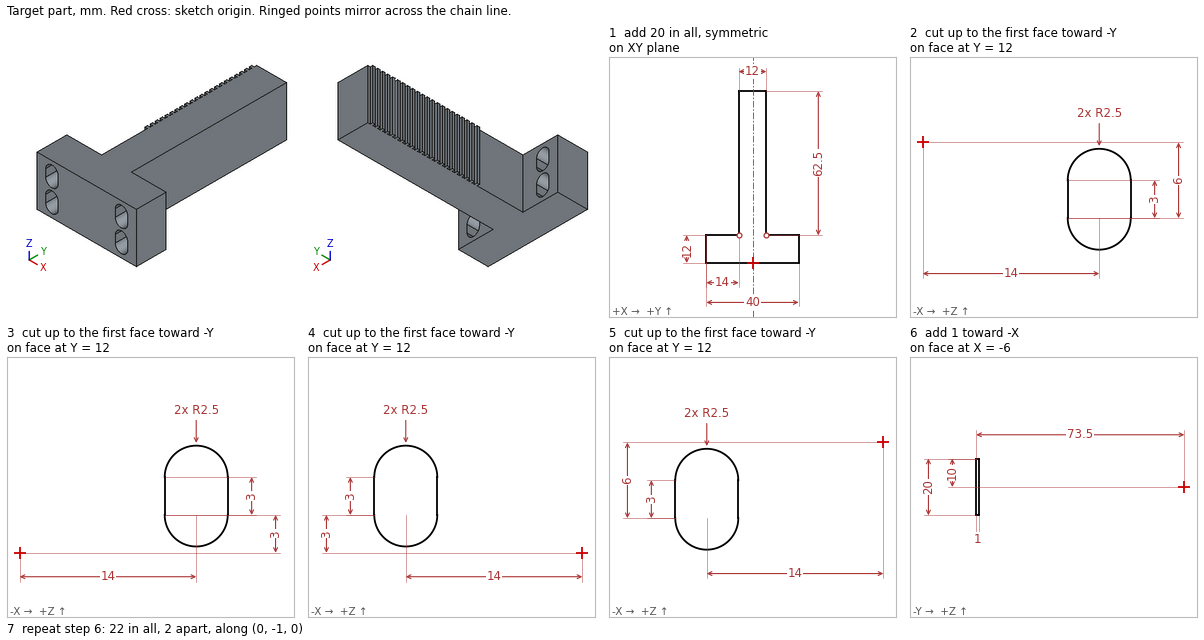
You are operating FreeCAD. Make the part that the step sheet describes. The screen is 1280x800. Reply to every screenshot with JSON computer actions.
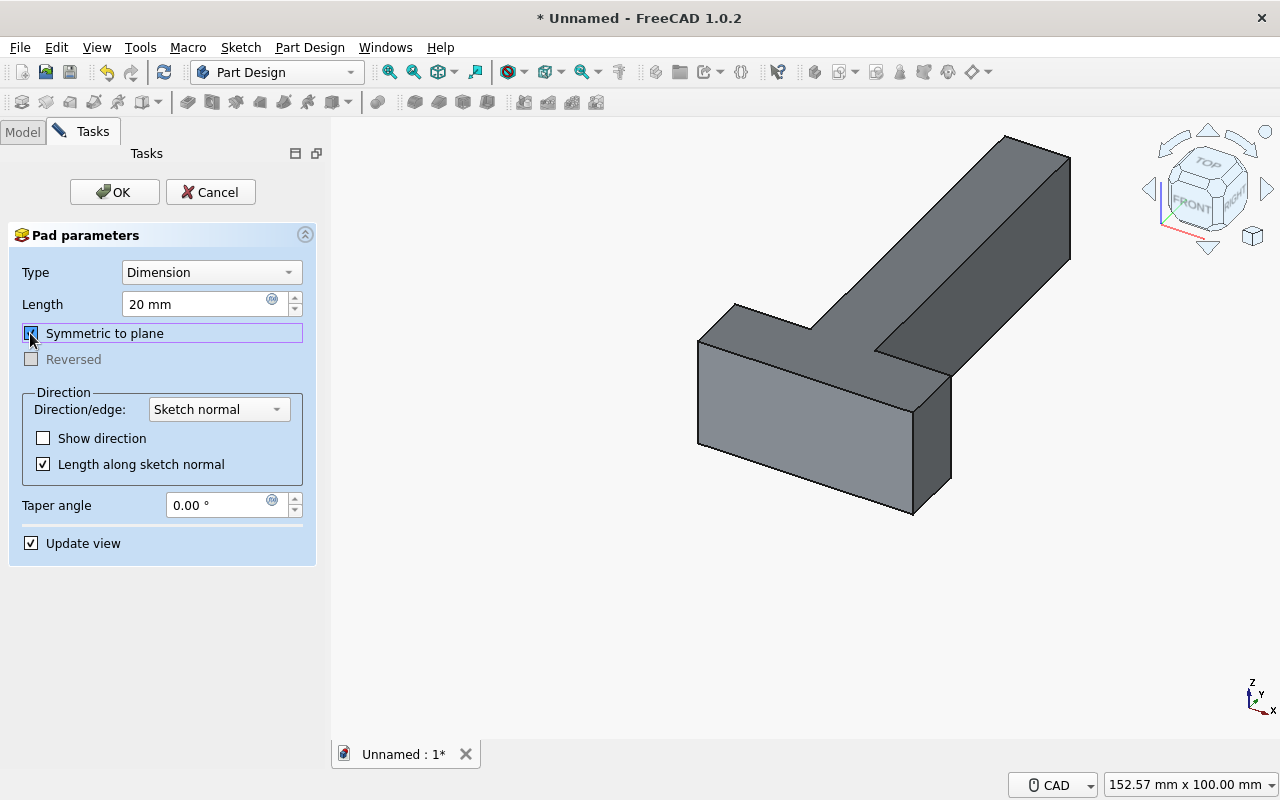
{"action": "left_click", "coordinate": [115, 192]}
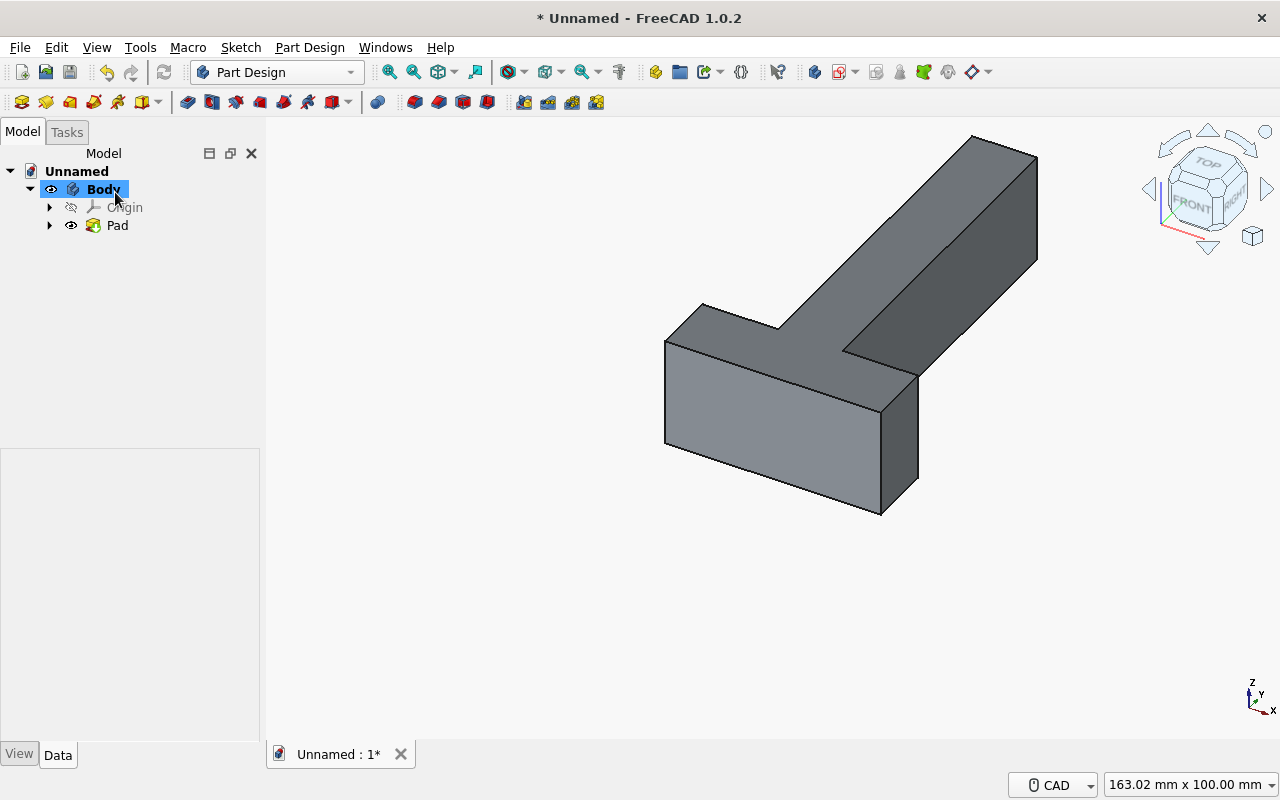
{"action": "left_click", "coordinate": [390, 72]}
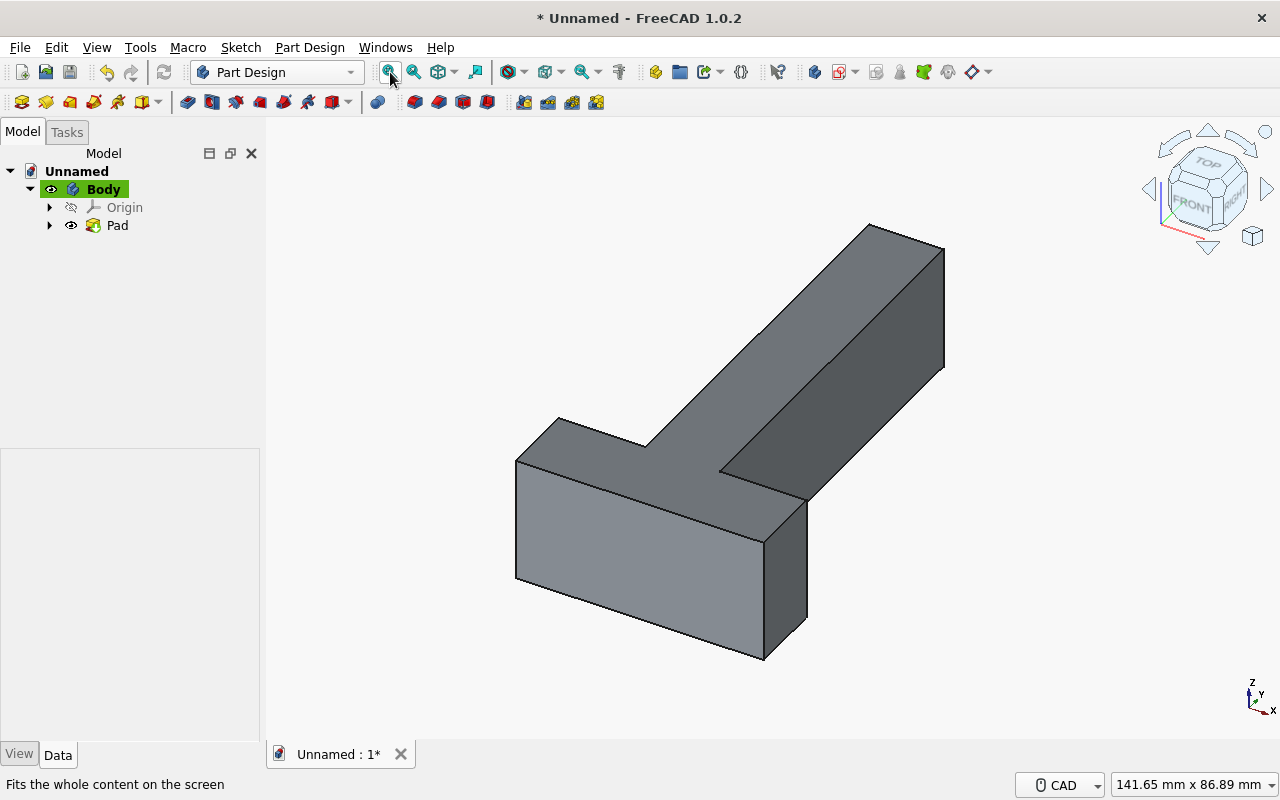
{"action": "key", "text": "4"}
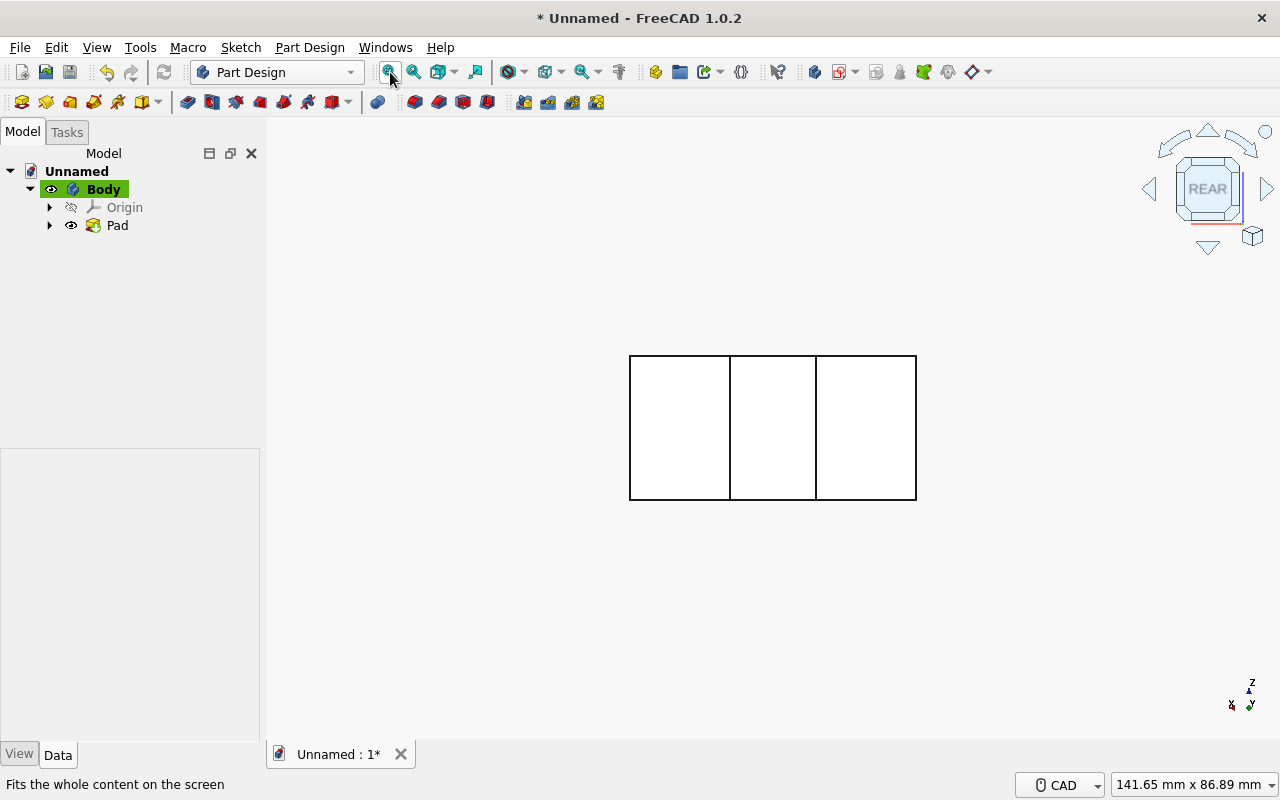
{"action": "left_click", "coordinate": [390, 72]}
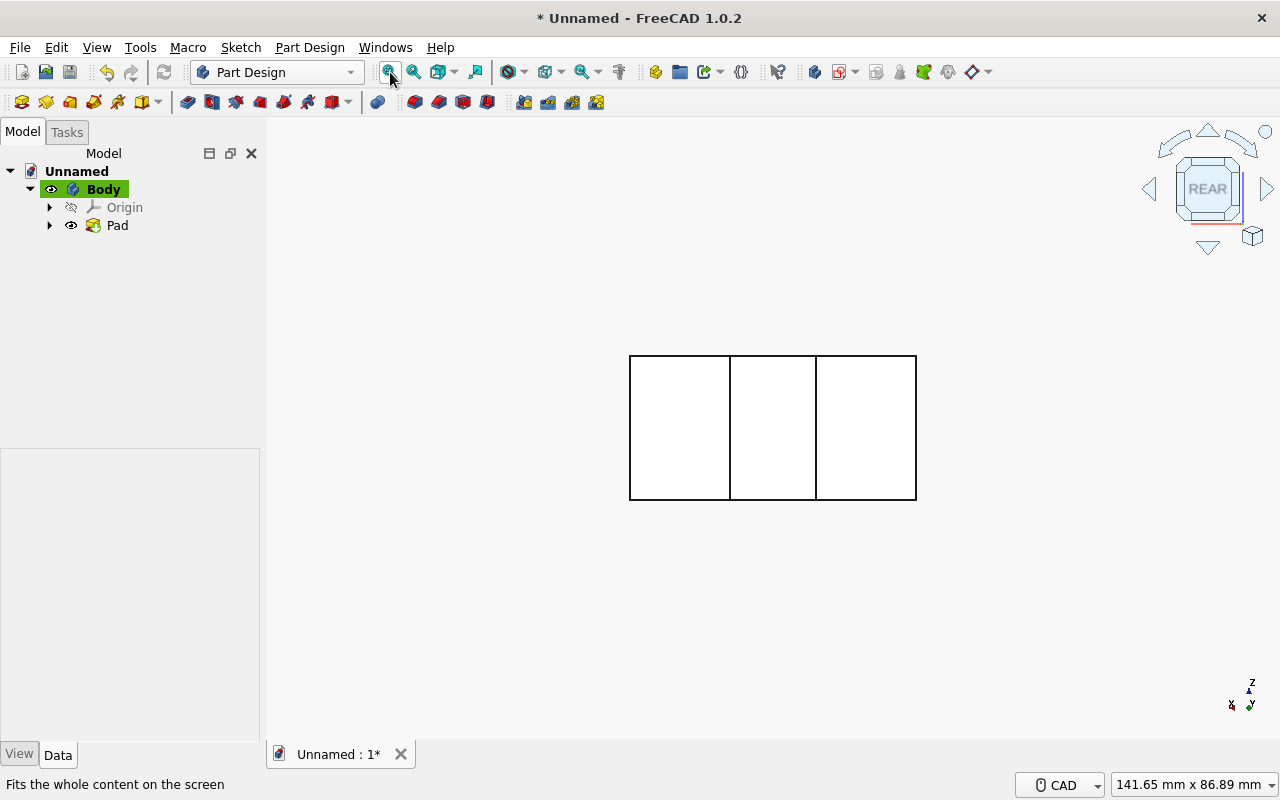
{"action": "left_click", "coordinate": [680, 407]}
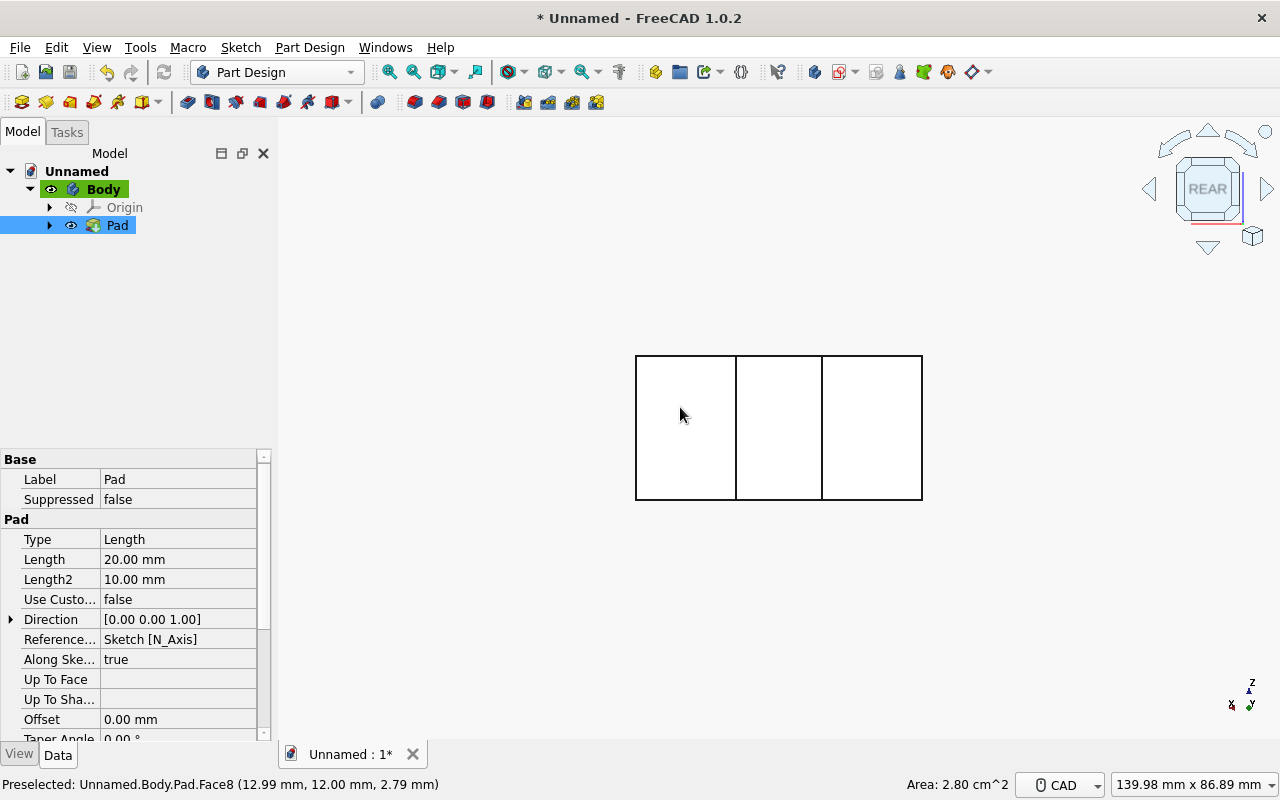
{"action": "left_click", "coordinate": [840, 72]}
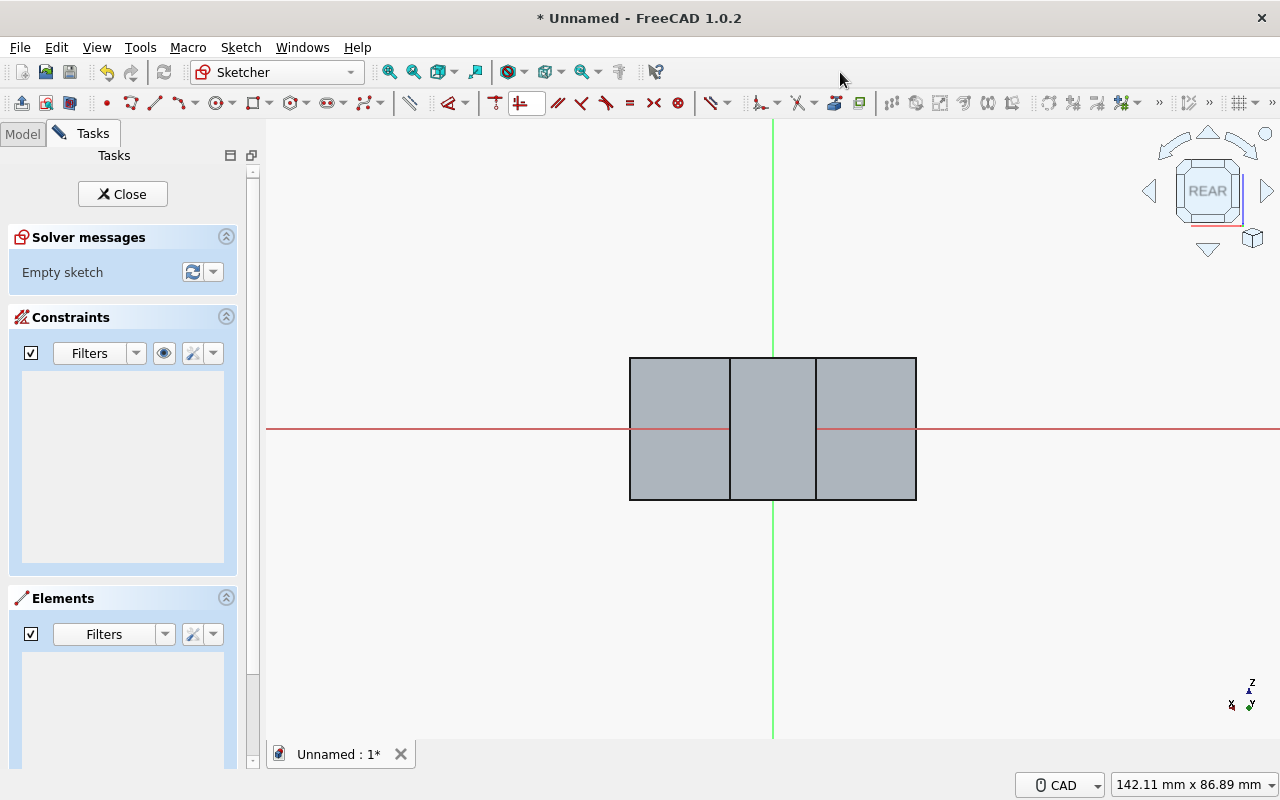
{"action": "scroll", "coordinate": [864, 467], "scroll_direction": "up", "scroll_amount": 8}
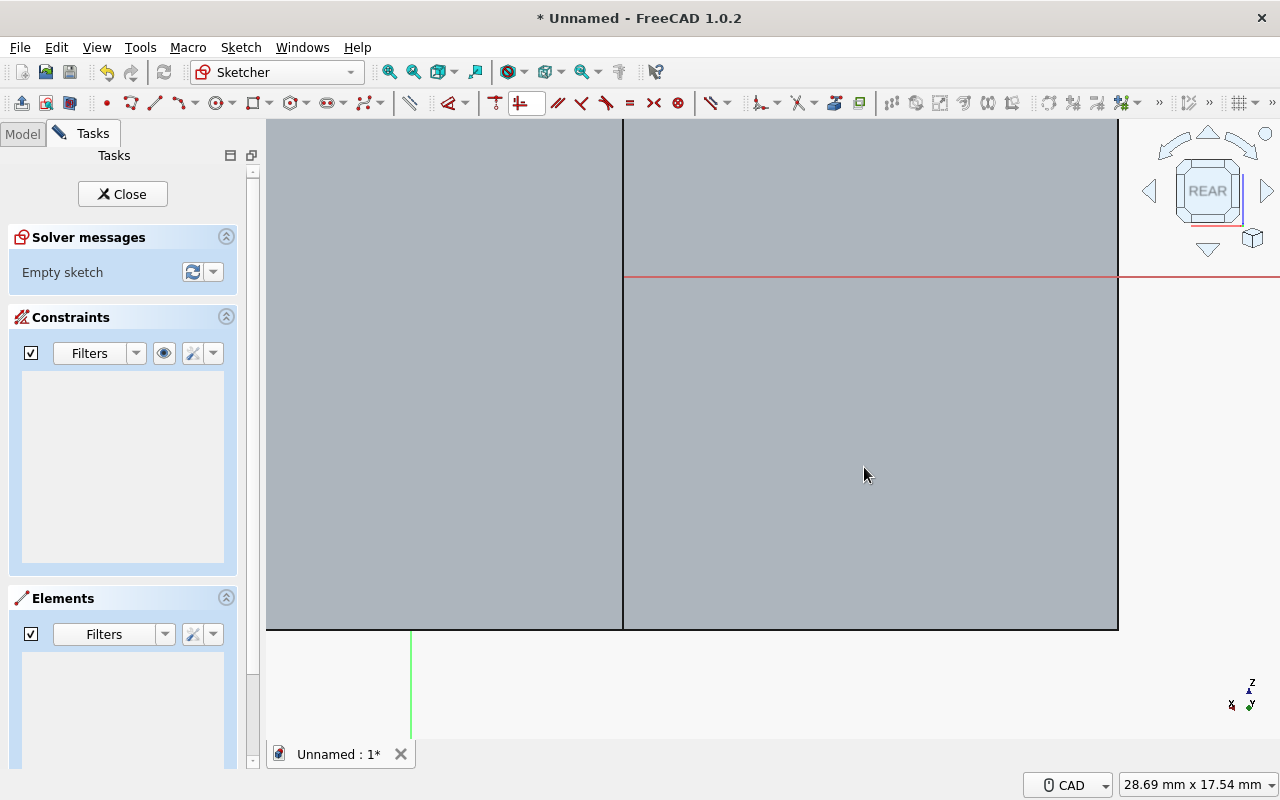
{"action": "left_click", "coordinate": [328, 104]}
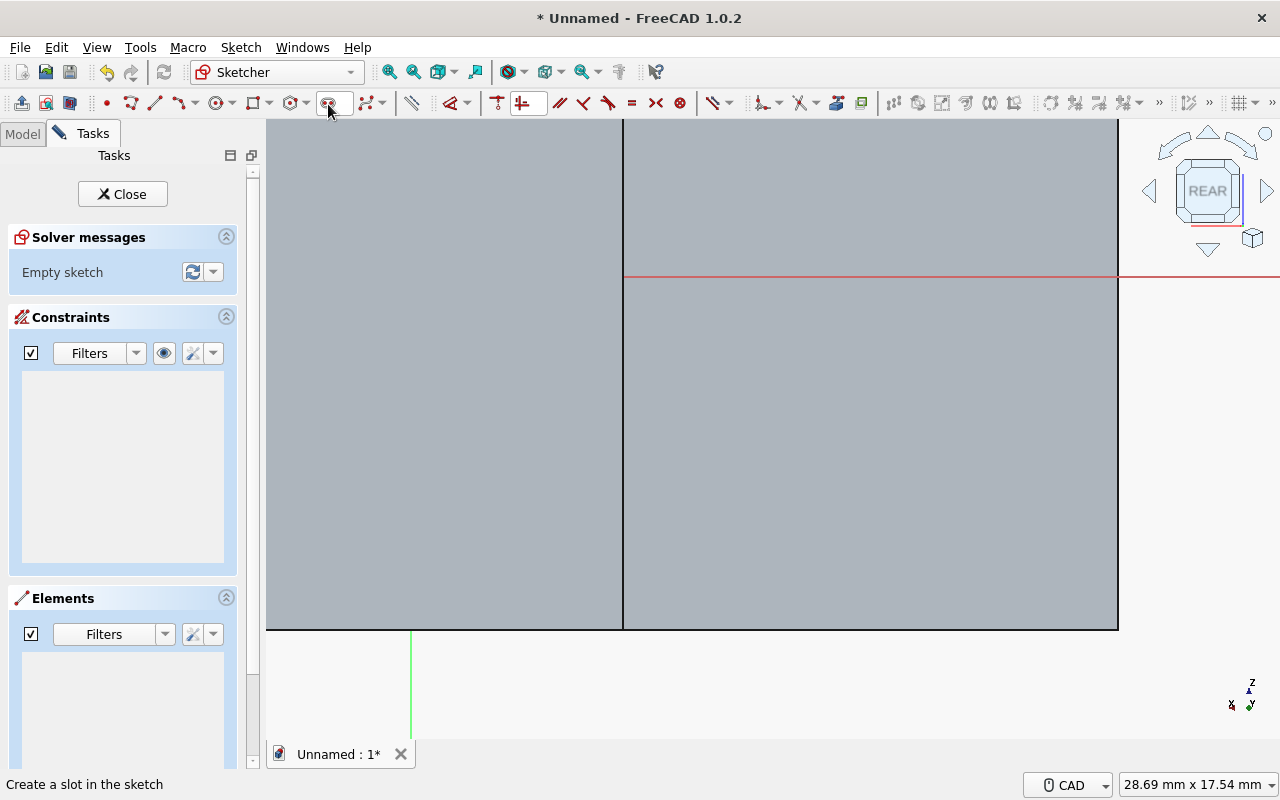
{"action": "left_click", "coordinate": [906, 489]}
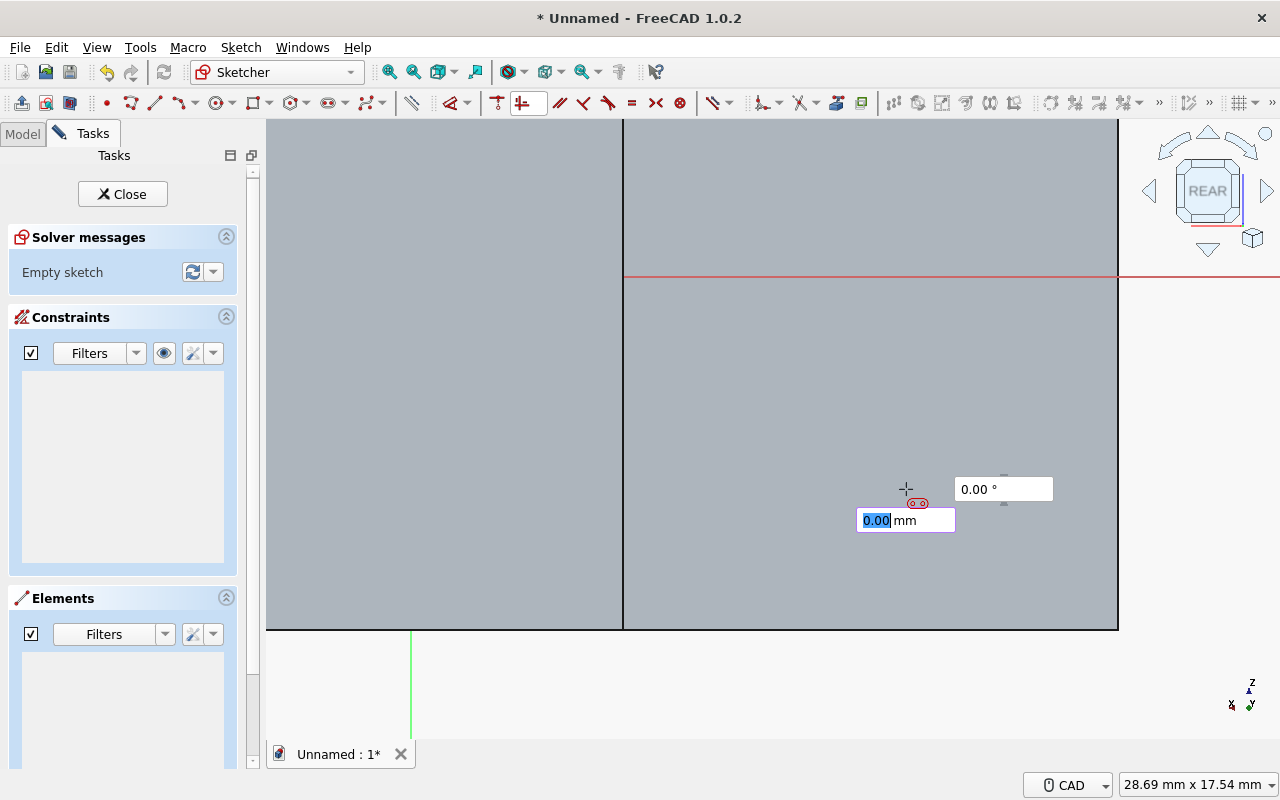
{"action": "left_click", "coordinate": [906, 383]}